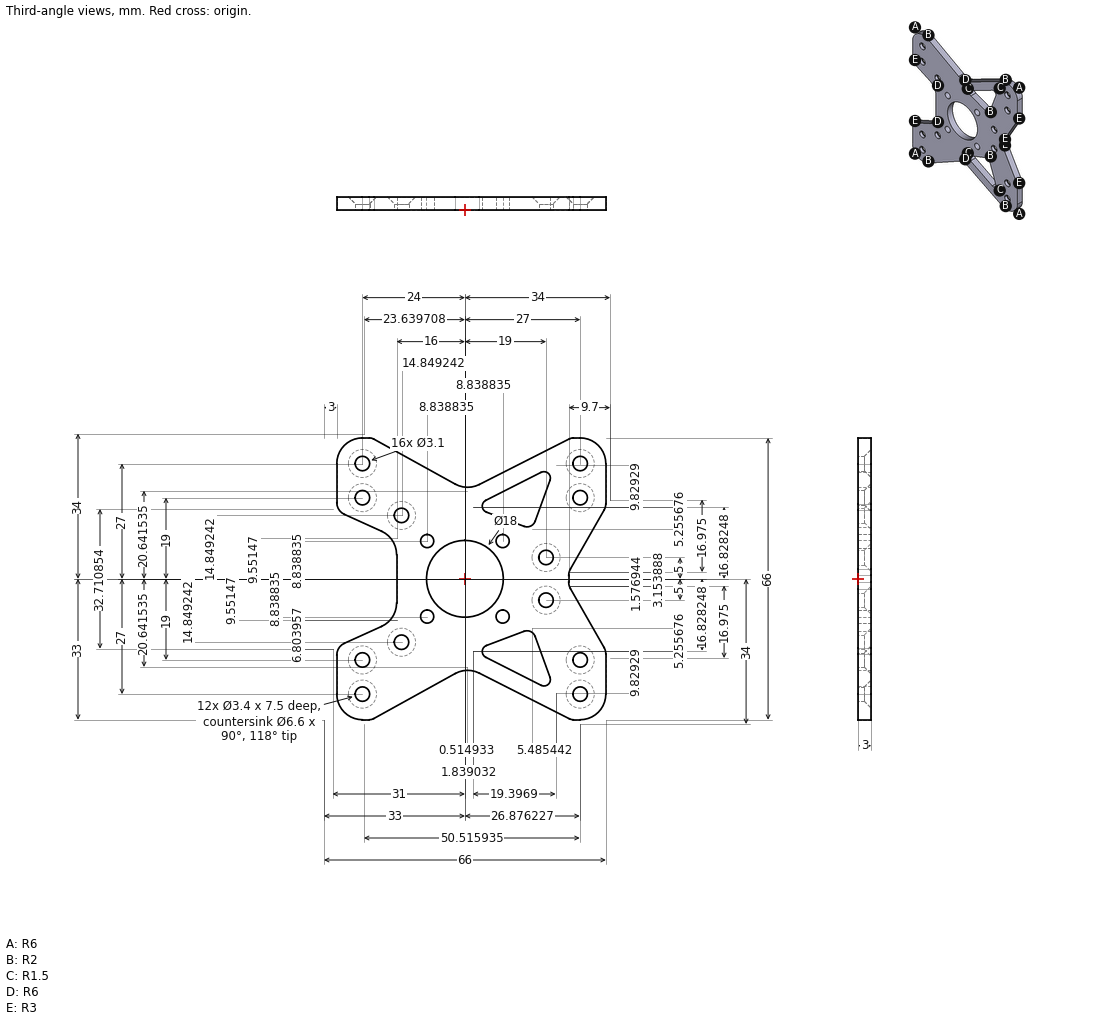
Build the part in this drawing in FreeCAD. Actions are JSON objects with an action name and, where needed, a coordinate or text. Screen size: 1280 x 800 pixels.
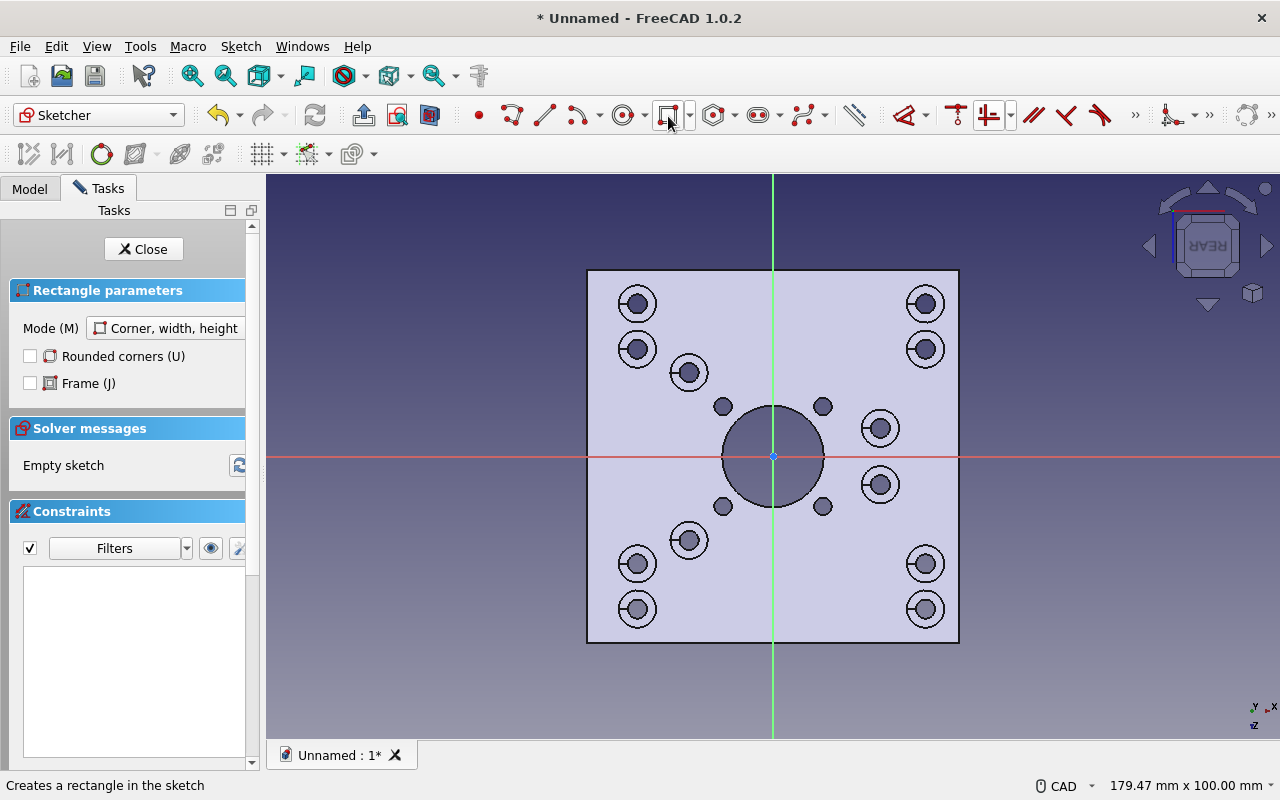
{"action": "left_click", "coordinate": [587, 270]}
{"action": "mouse_move", "coordinate": [603, 643]}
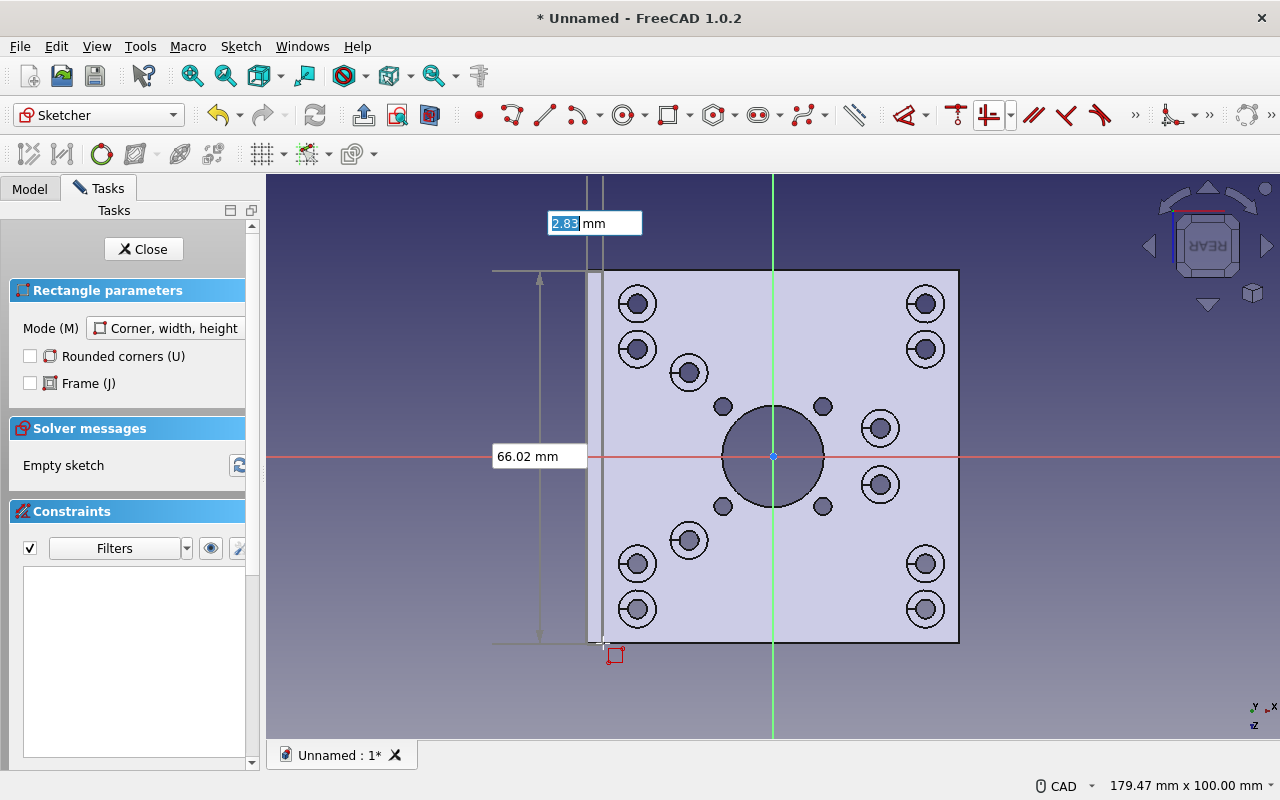
{"action": "type", "text": "3"}
{"action": "key", "text": "Tab"}
{"action": "type", "text": "66"}
{"action": "key", "text": "Return"}
{"action": "key", "text": "Escape"}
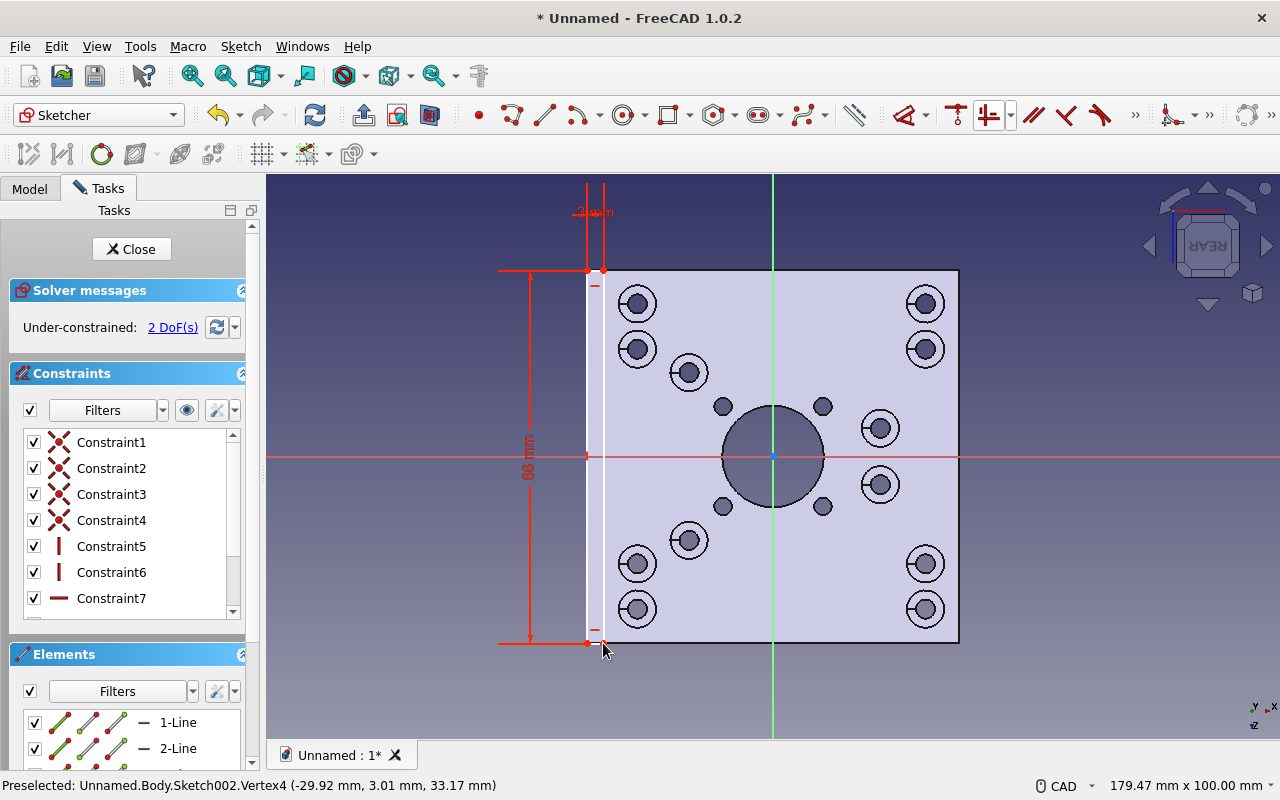
{"action": "left_click", "coordinate": [904, 116]}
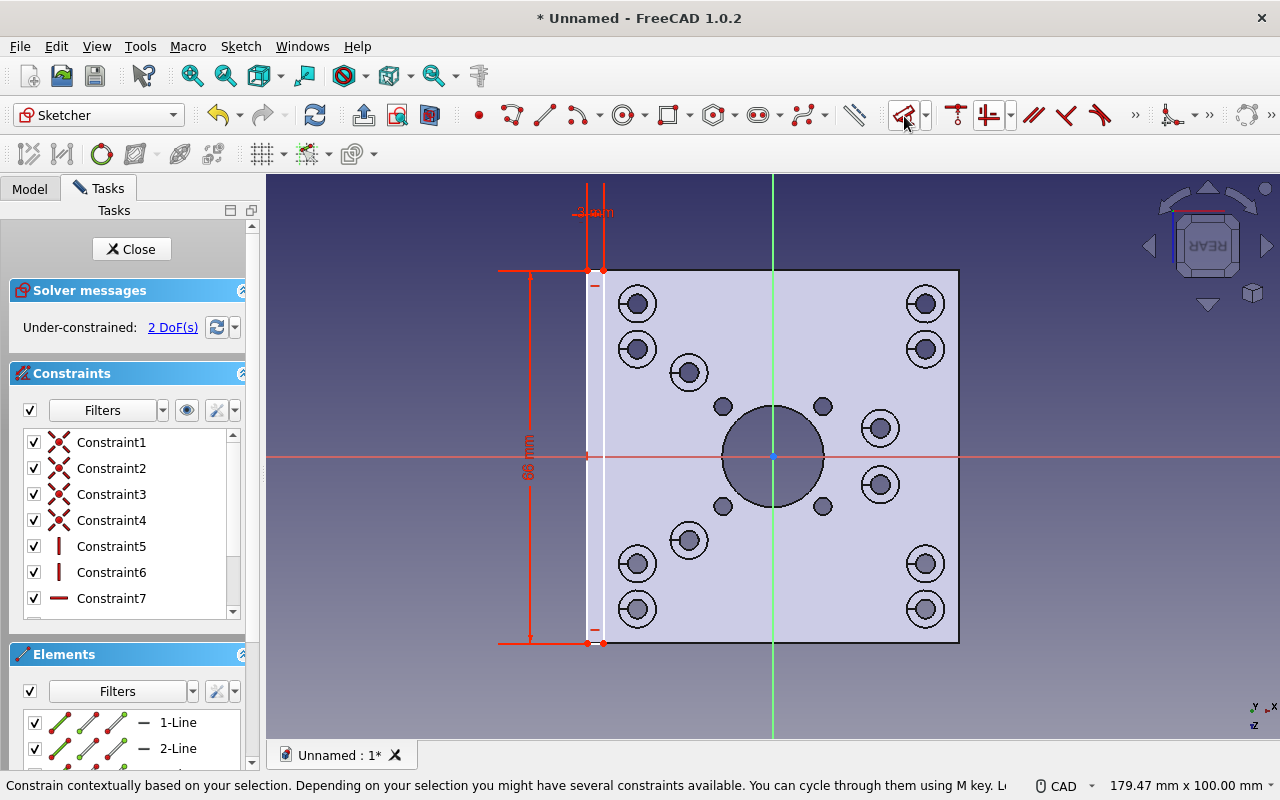
{"action": "left_click", "coordinate": [587, 271]}
{"action": "left_click", "coordinate": [680, 237]}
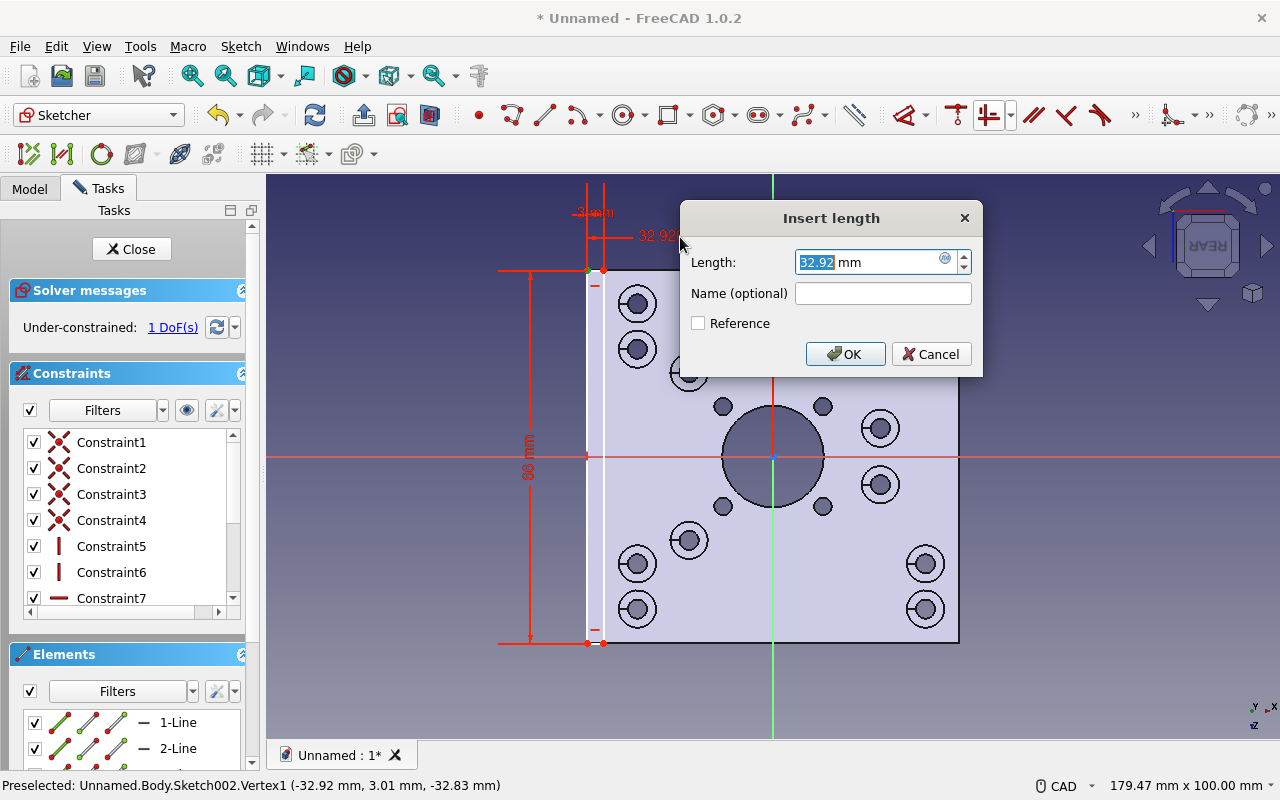
{"action": "type", "text": "33"}
{"action": "key", "text": "Return"}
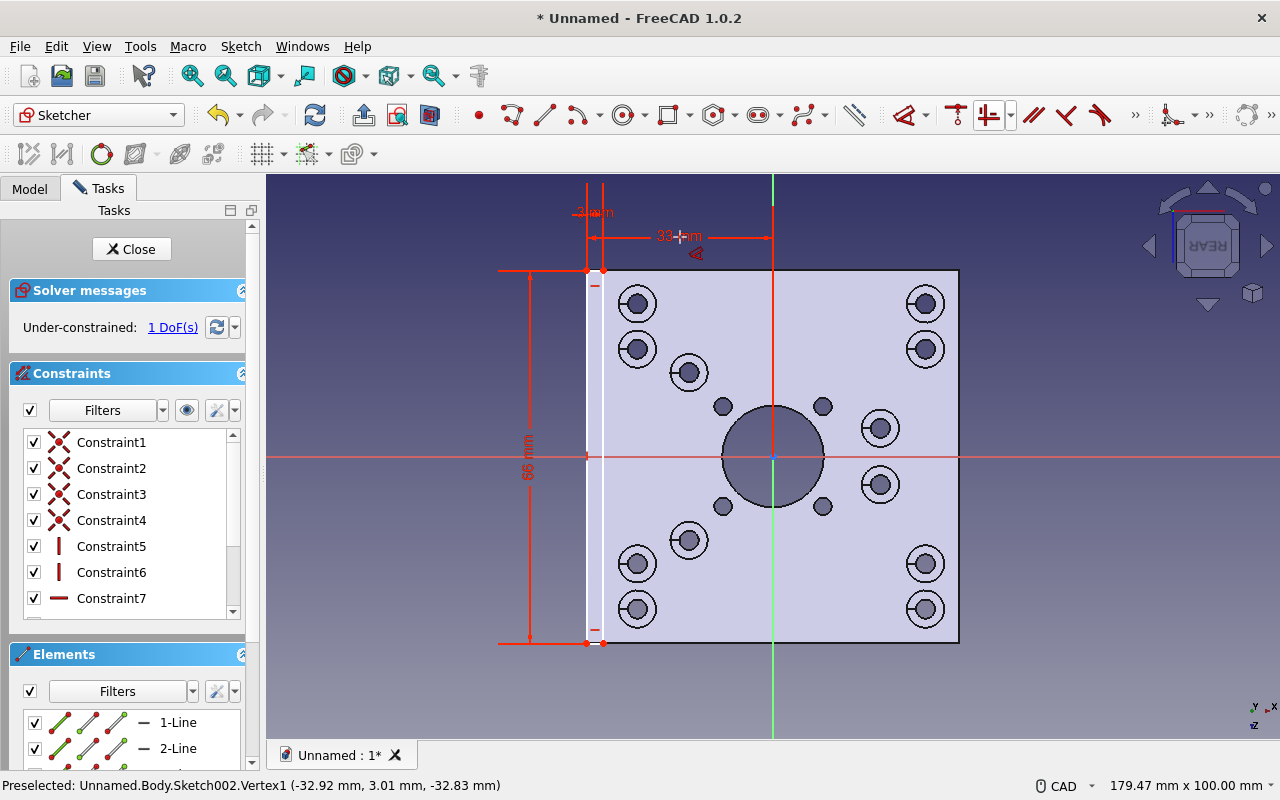
{"action": "left_click", "coordinate": [587, 271]}
{"action": "left_click", "coordinate": [807, 364]}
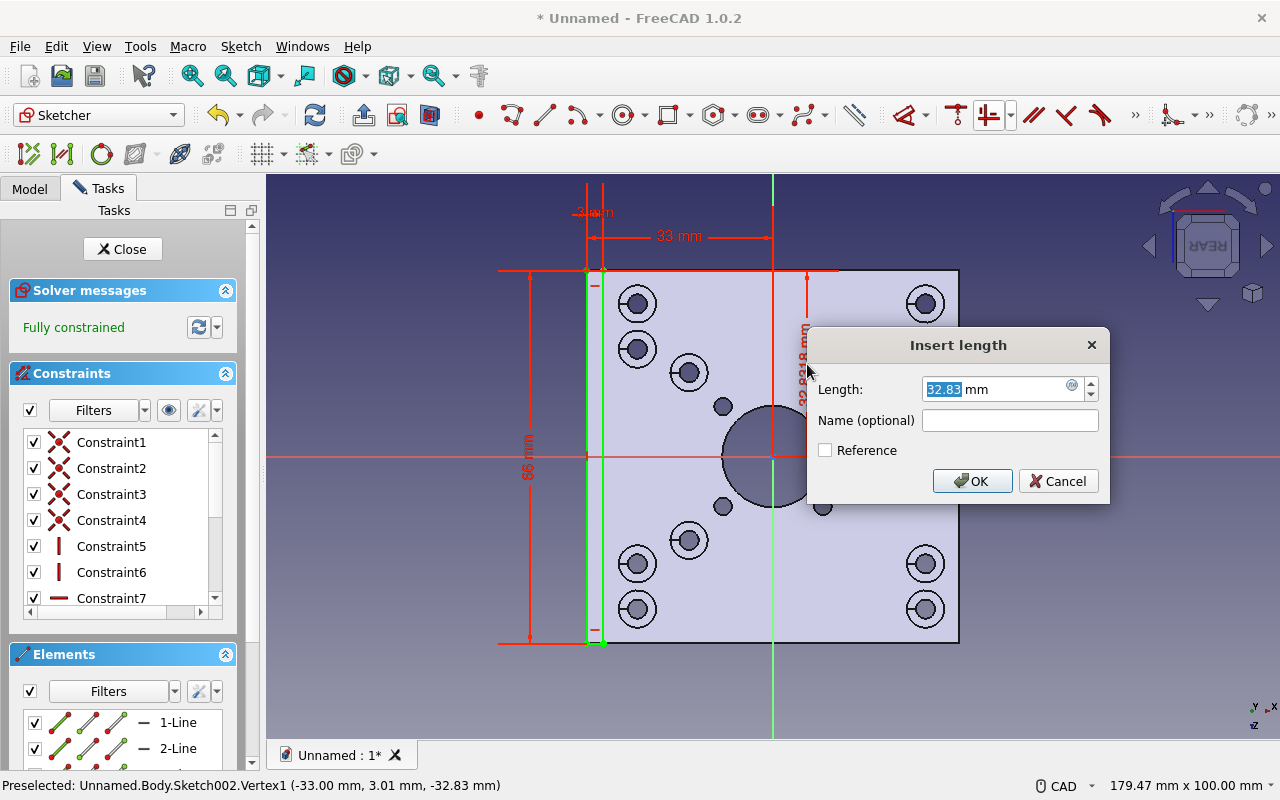
{"action": "type", "text": "33"}
{"action": "key", "text": "Return"}
{"action": "key", "text": "Escape"}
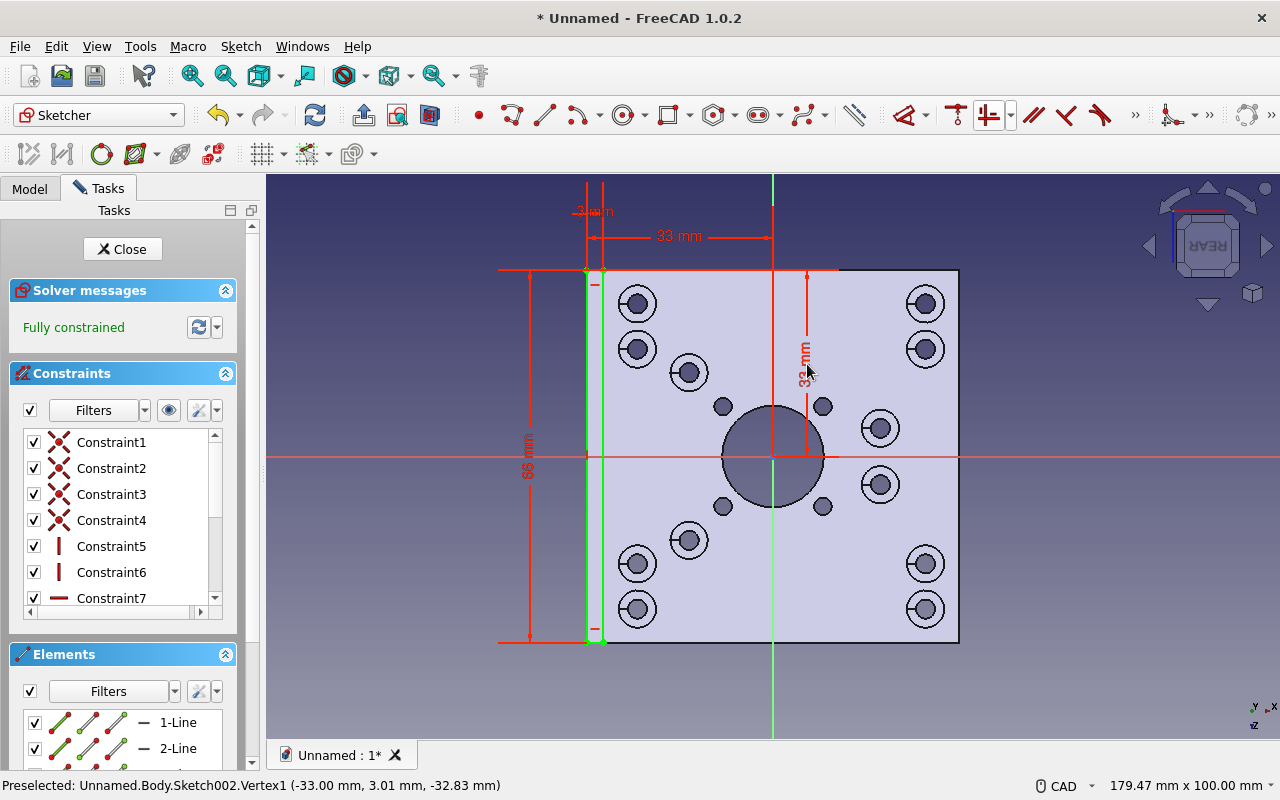
{"action": "left_click", "coordinate": [123, 249]}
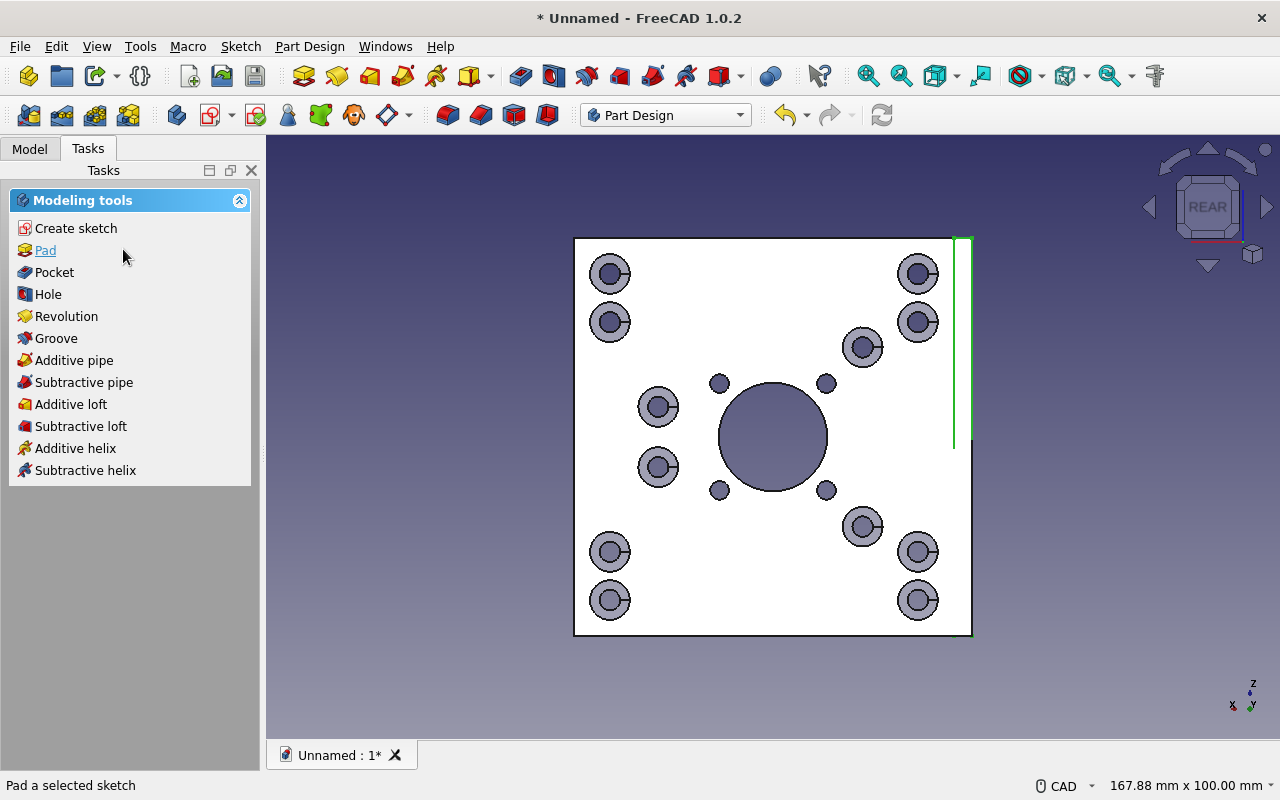
{"action": "left_click", "coordinate": [521, 76]}